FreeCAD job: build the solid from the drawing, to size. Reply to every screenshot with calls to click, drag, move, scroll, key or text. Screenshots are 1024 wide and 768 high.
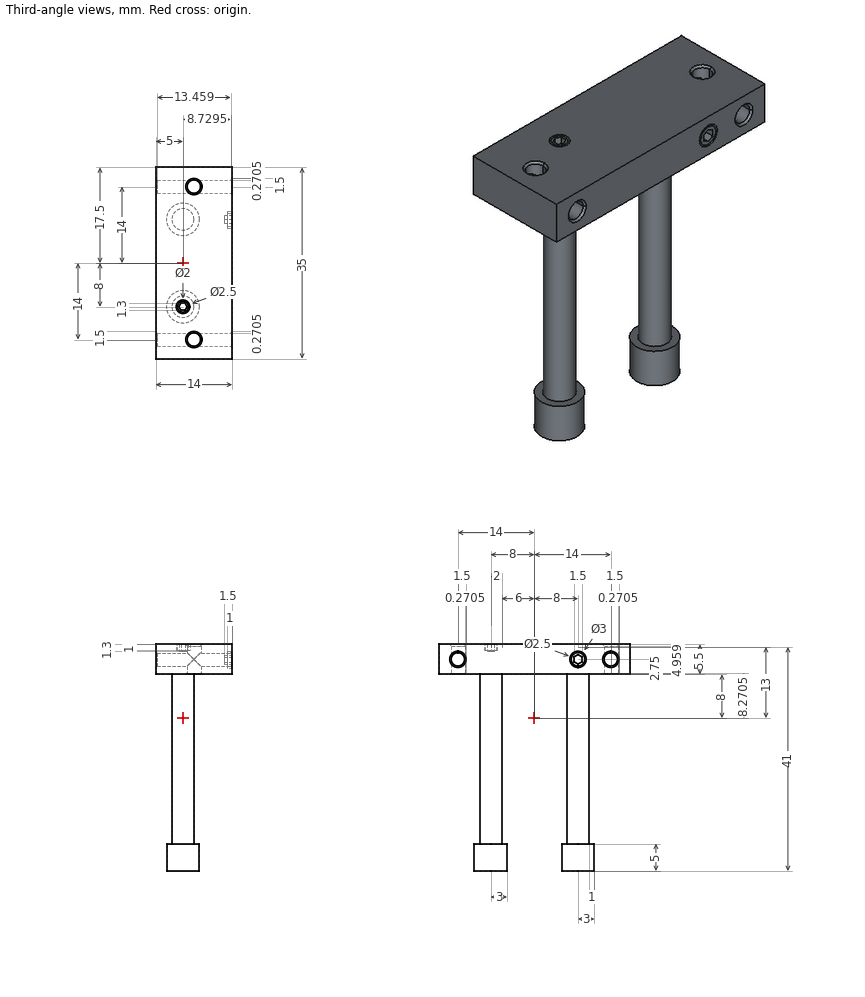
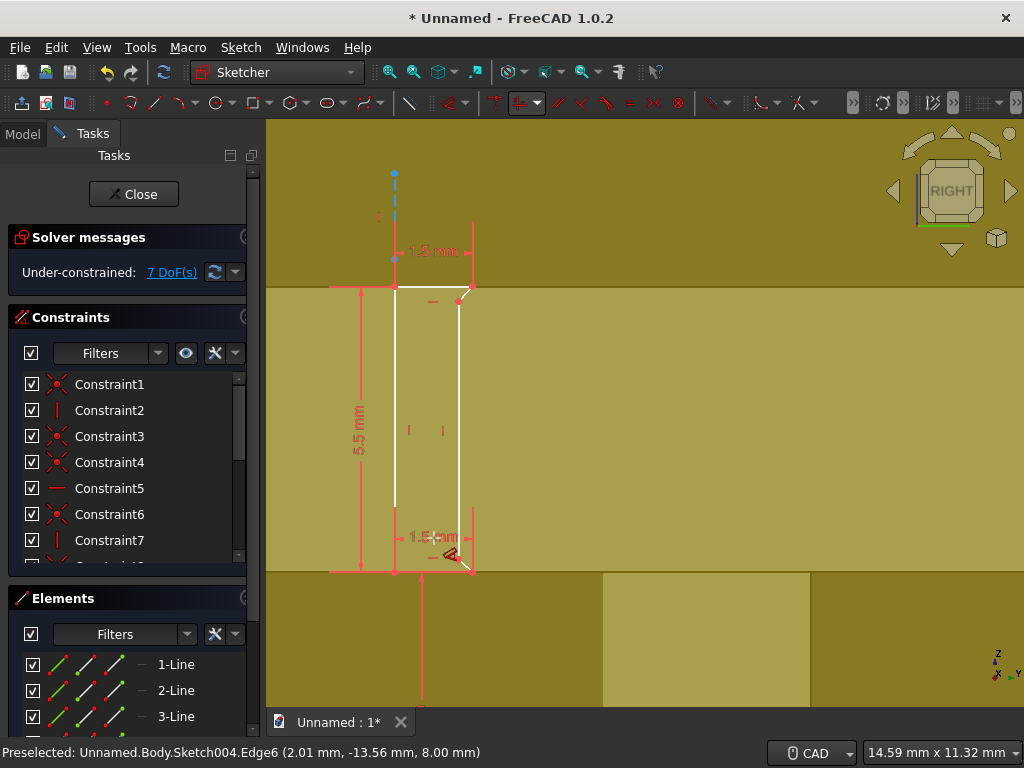
click(395, 287)
click(627, 253)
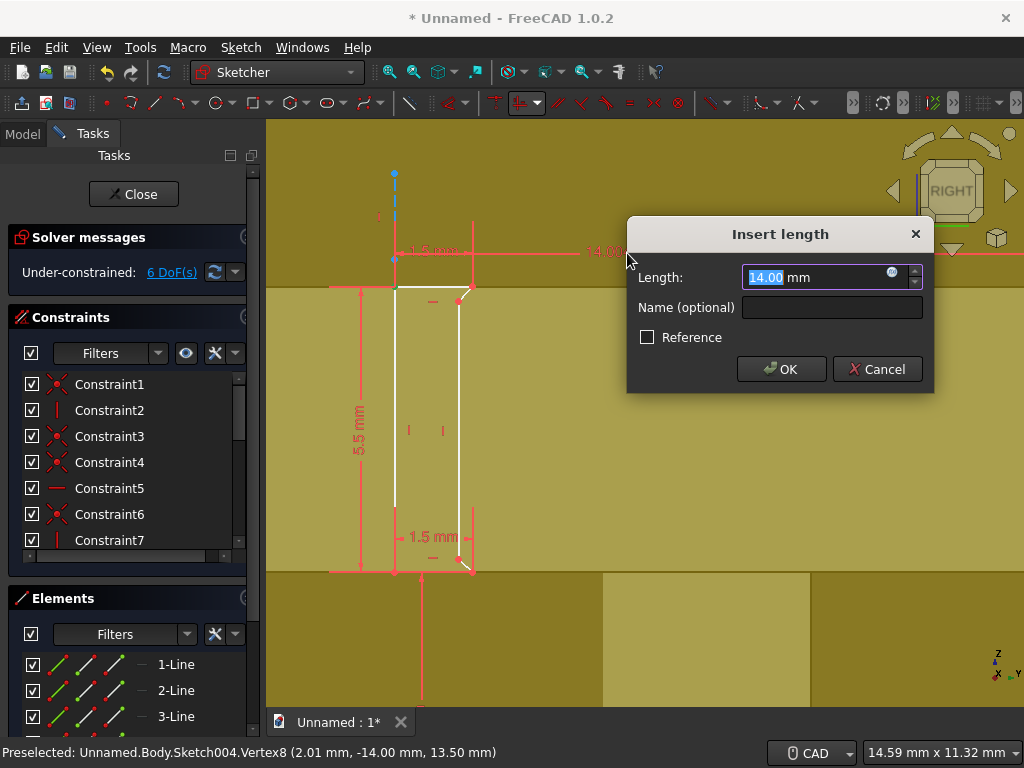
text(14)
key(Return)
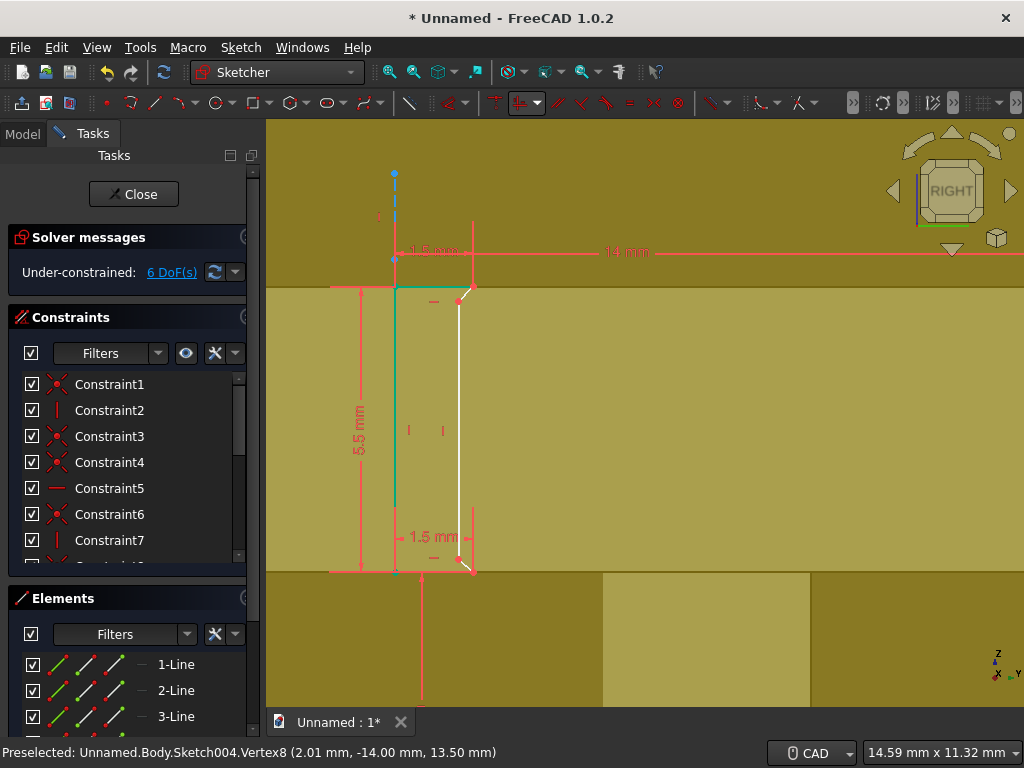
click(395, 259)
click(627, 225)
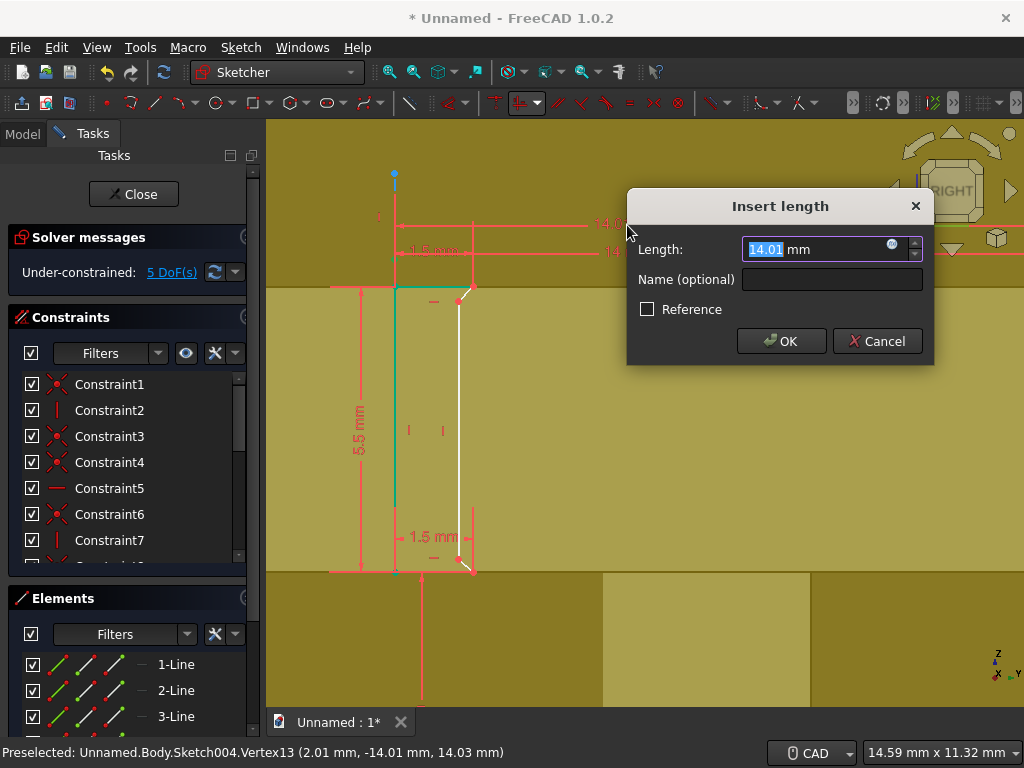
text(14)
key(Return)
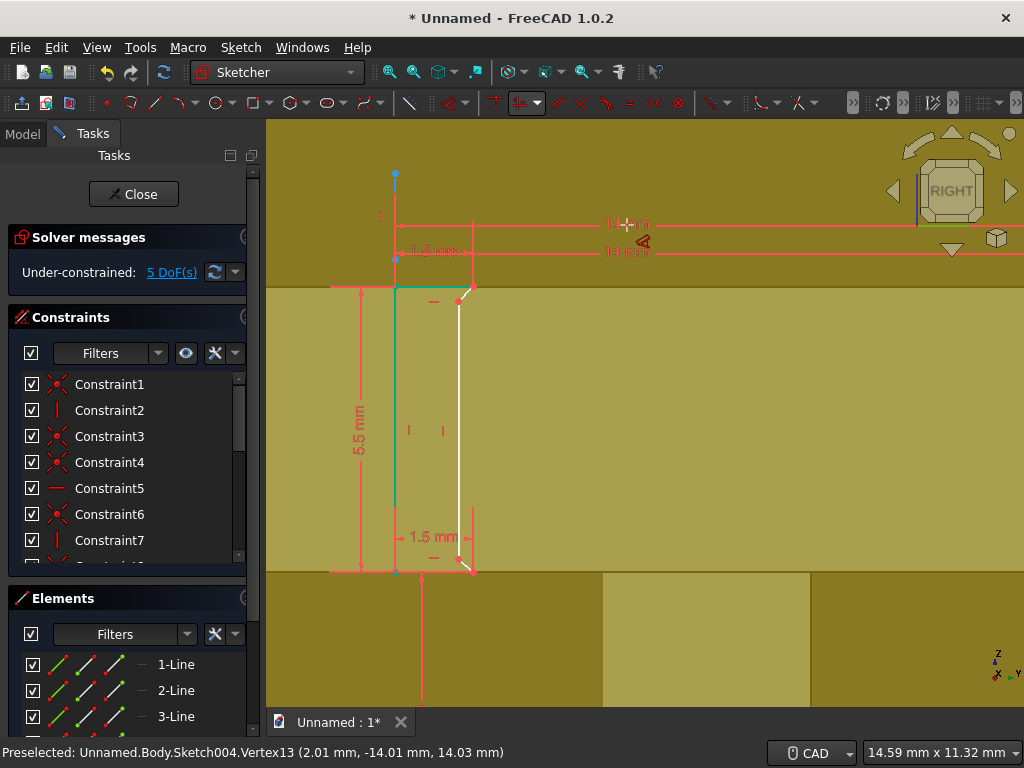
click(459, 482)
click(425, 371)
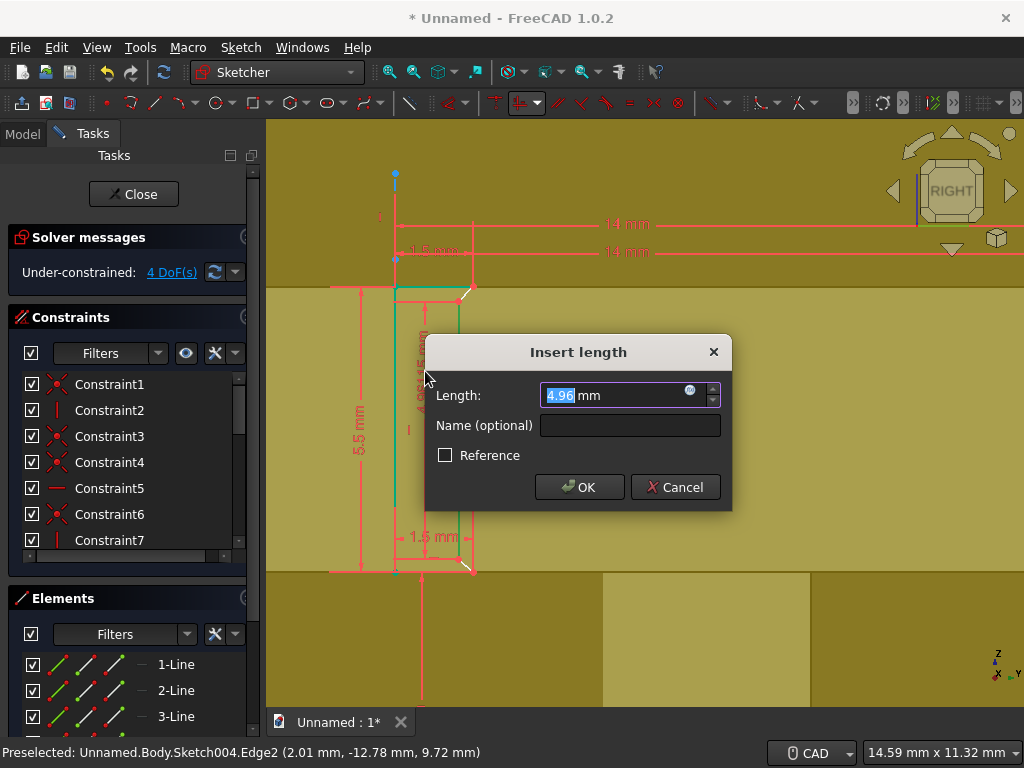
text(4.959)
key(Return)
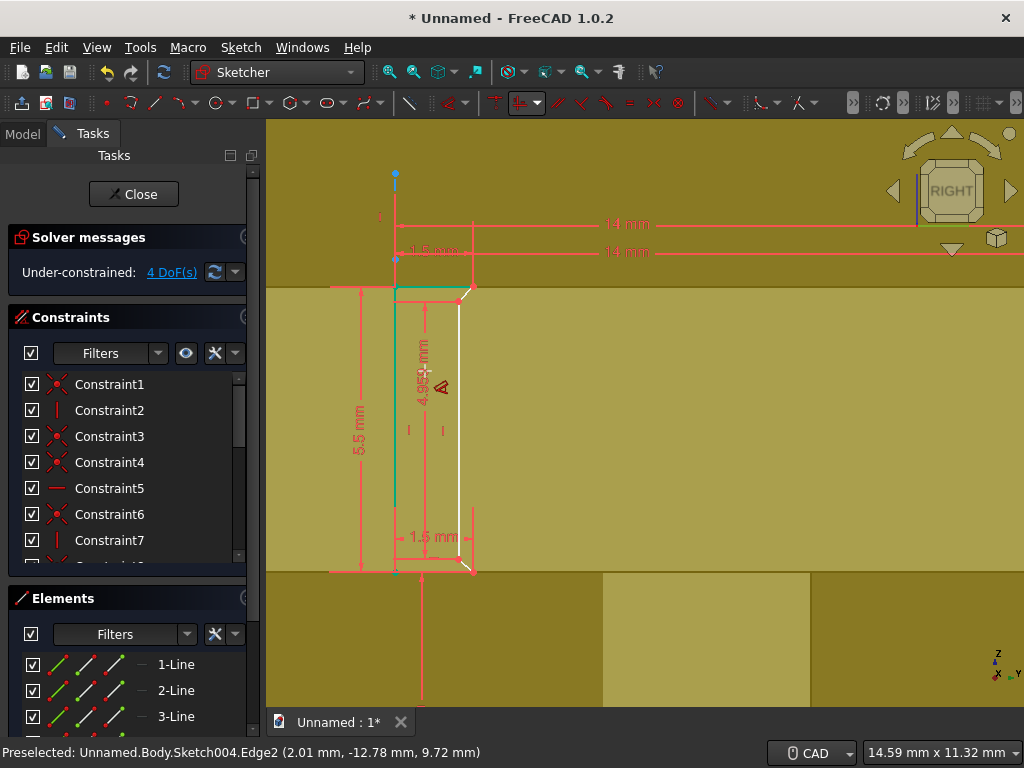
click(459, 559)
click(425, 619)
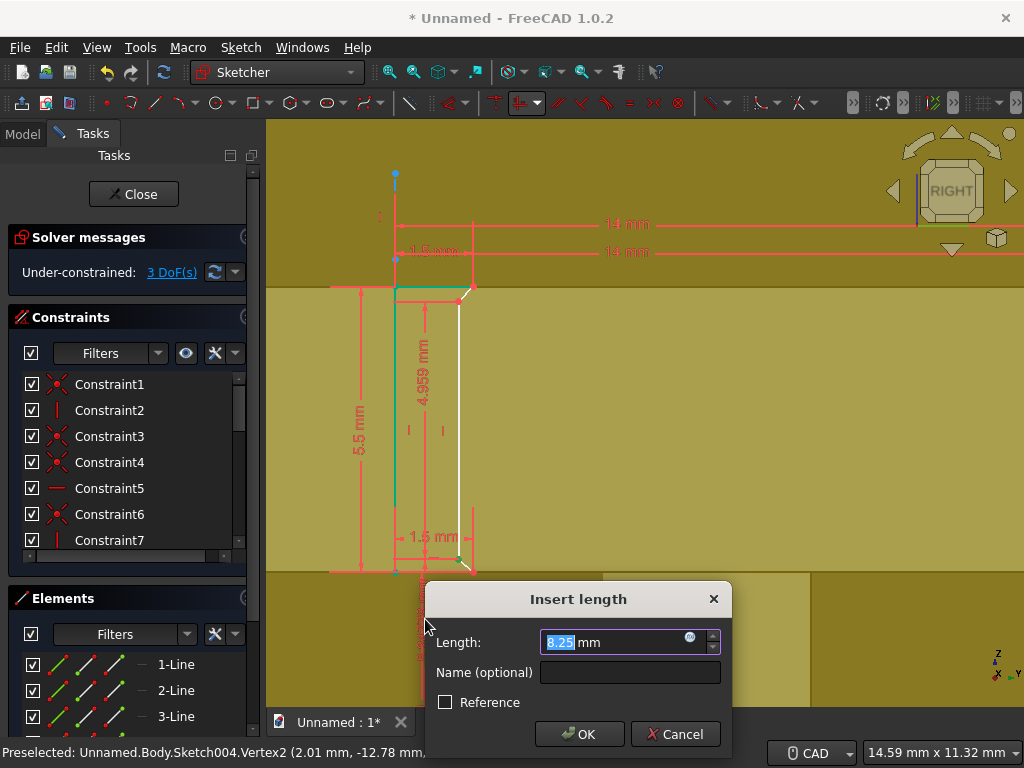
text(8.2705)
key(Return)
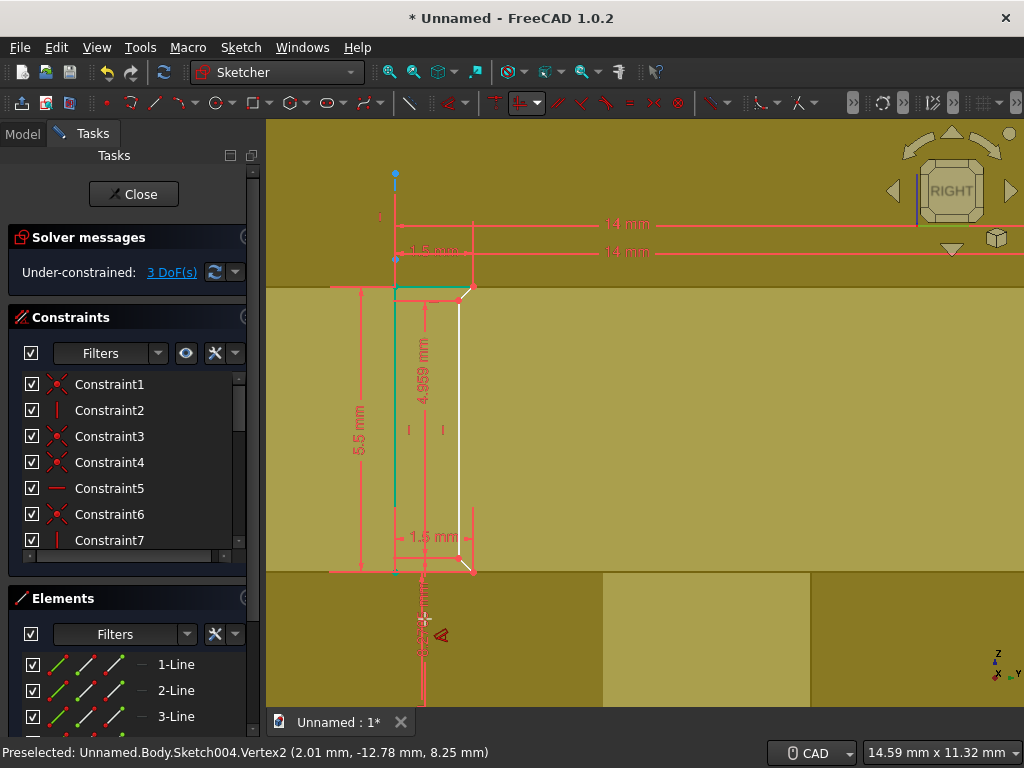
scroll(464, 564, up, 6)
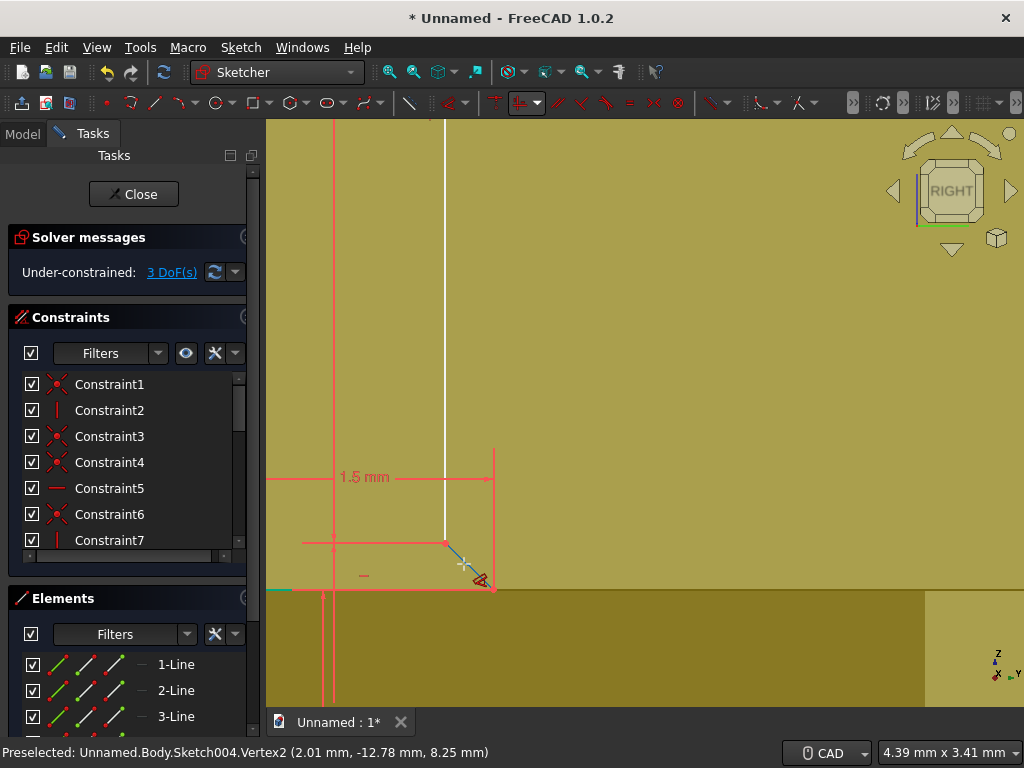
click(465, 562)
click(469, 509)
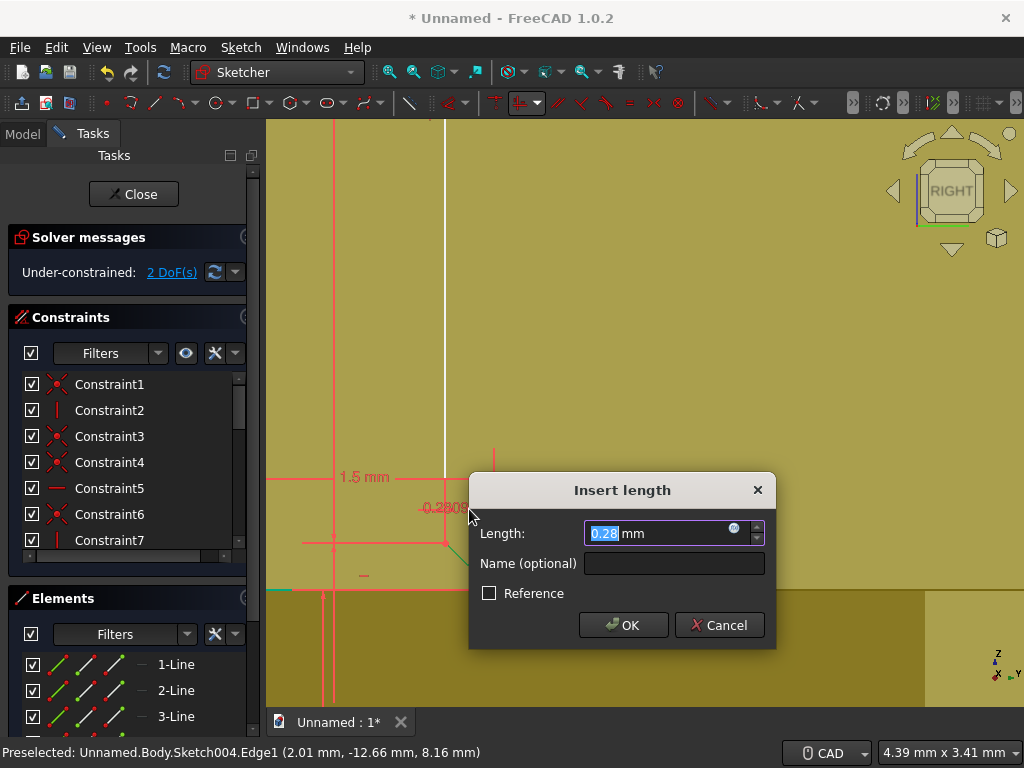
text(0.2705)
key(Return)
key(Escape)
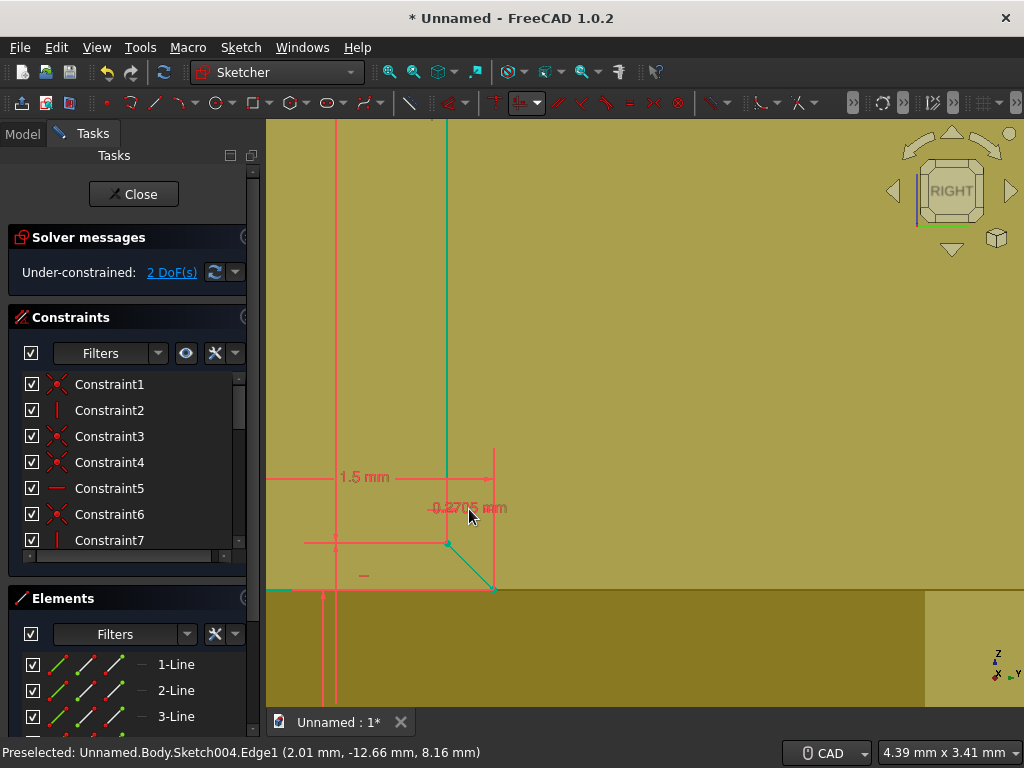
click(134, 194)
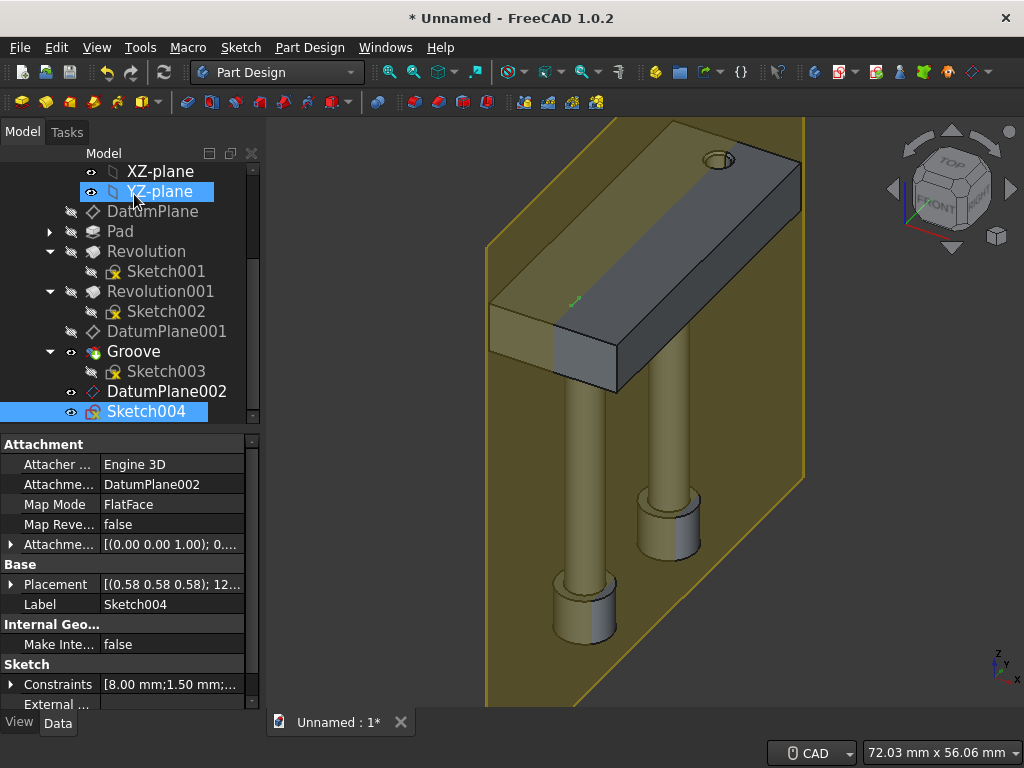
click(236, 102)